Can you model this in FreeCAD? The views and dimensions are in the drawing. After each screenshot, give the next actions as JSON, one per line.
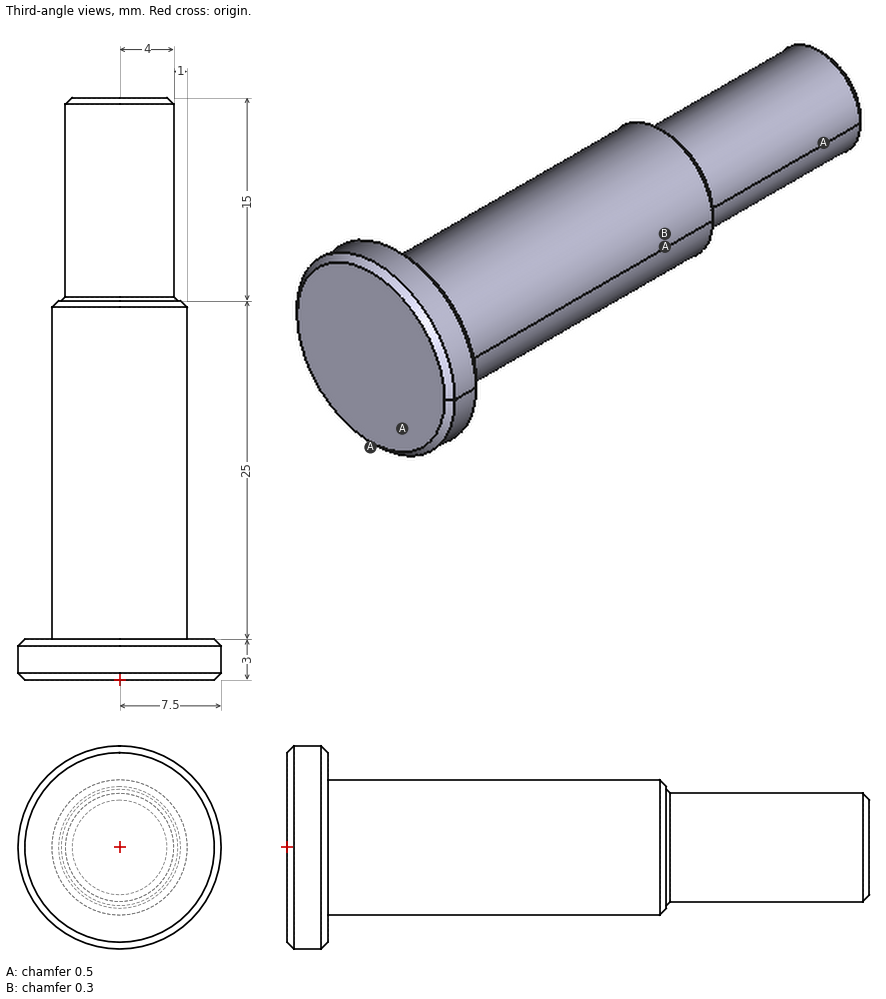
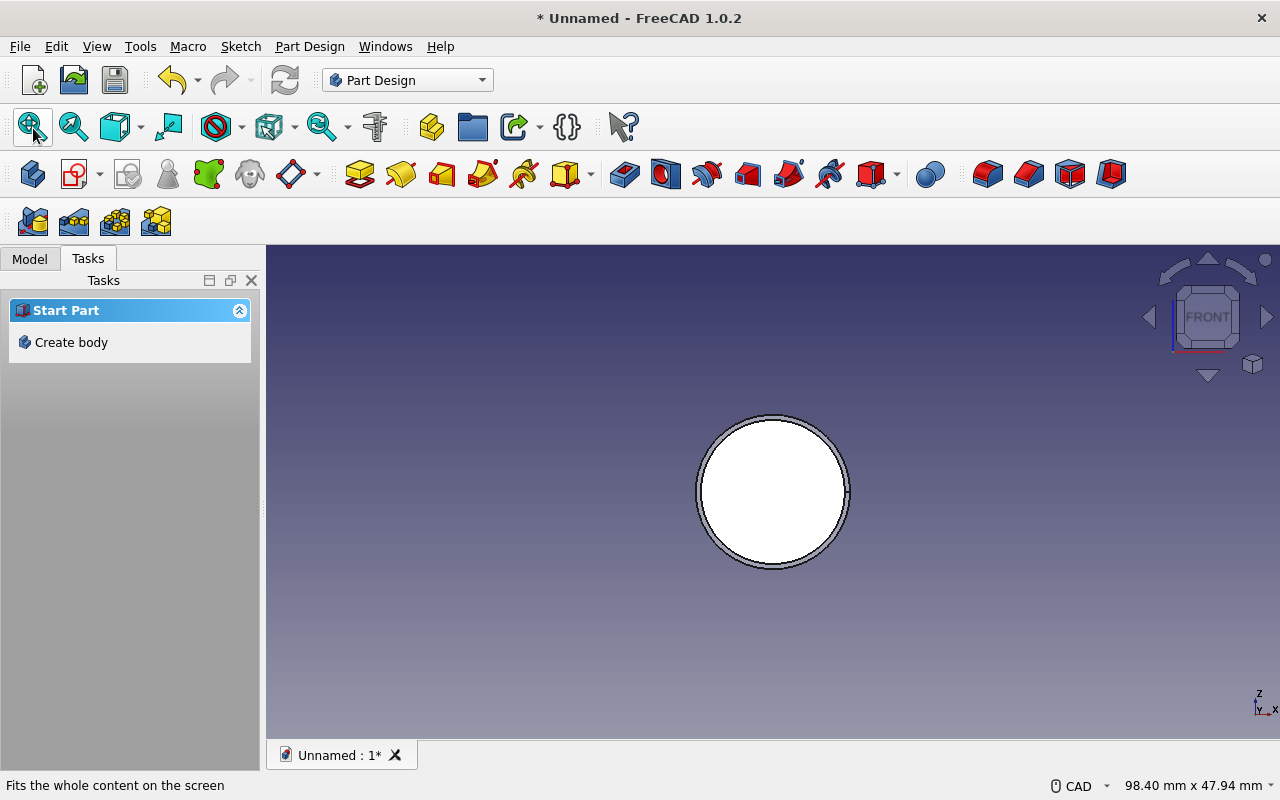
{"action": "key", "text": "3"}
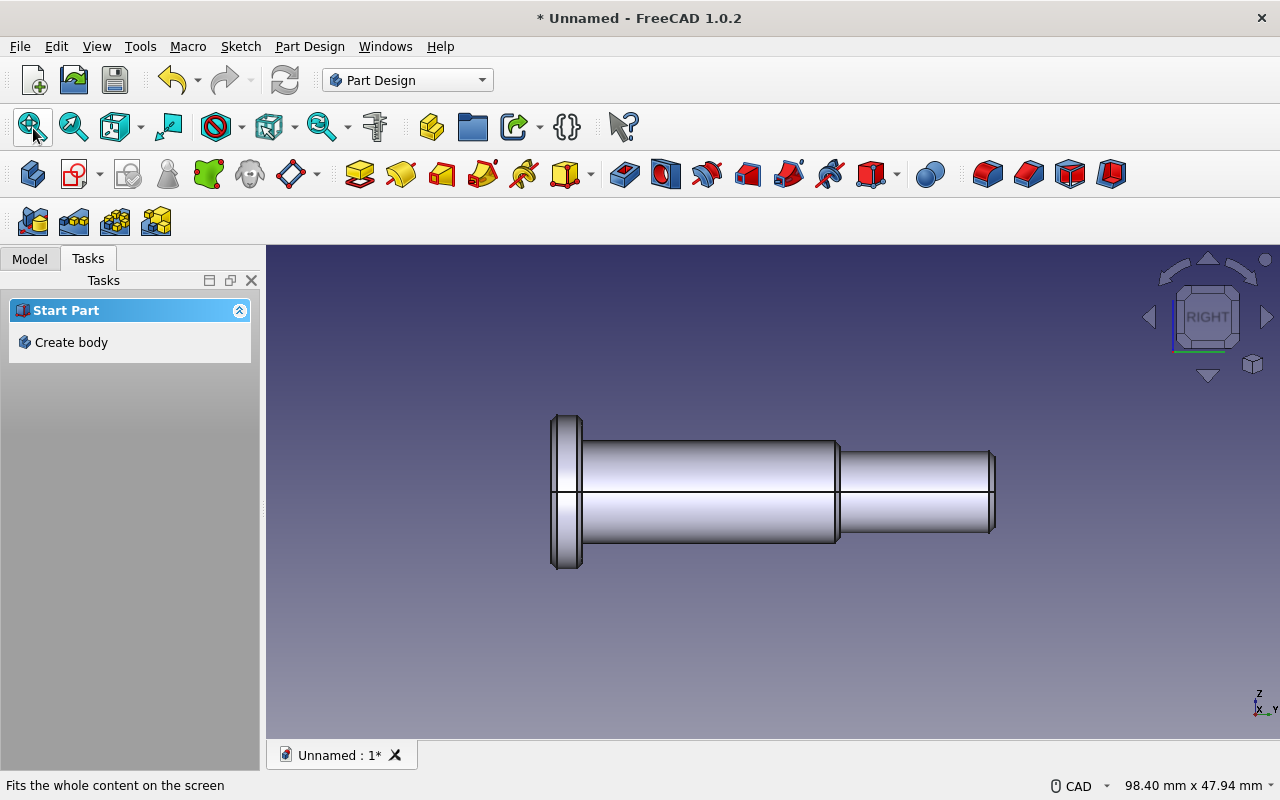
{"action": "left_click", "coordinate": [33, 128]}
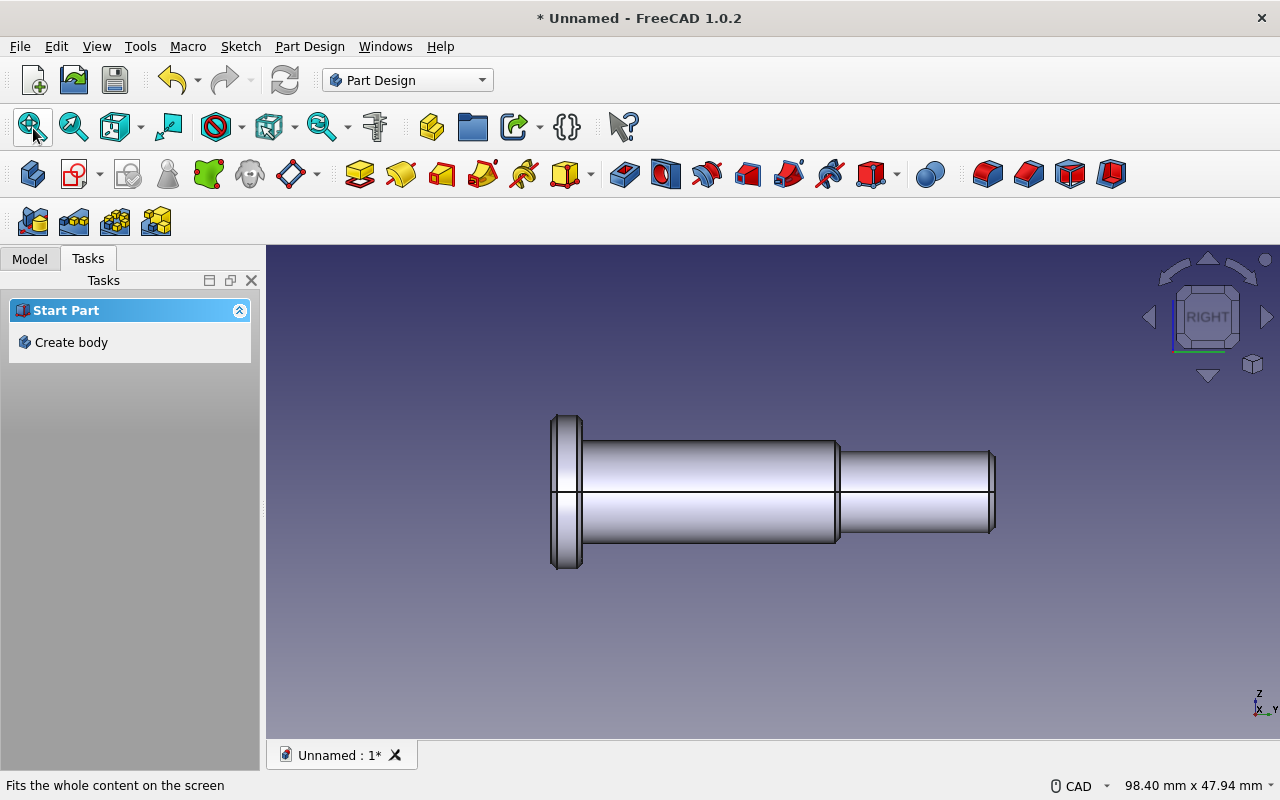
{"action": "key", "text": "5"}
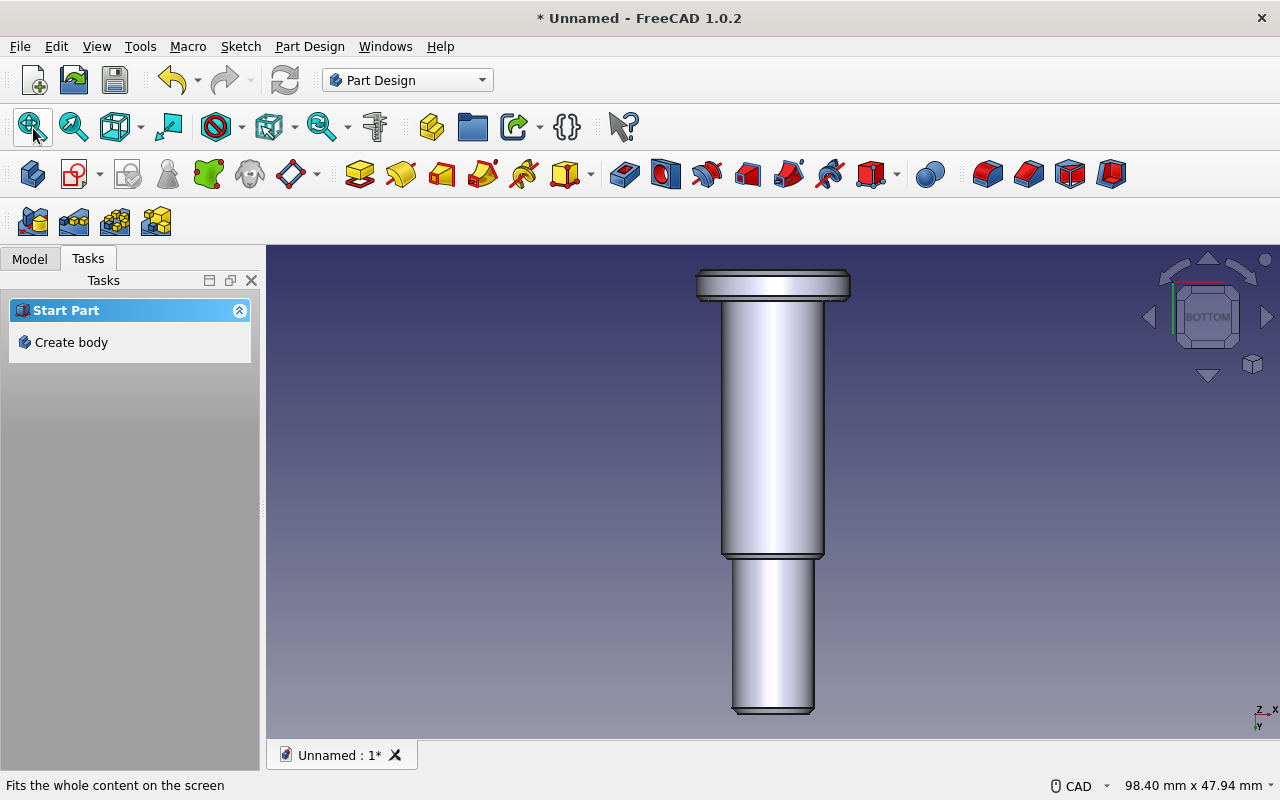
{"action": "key", "text": "4"}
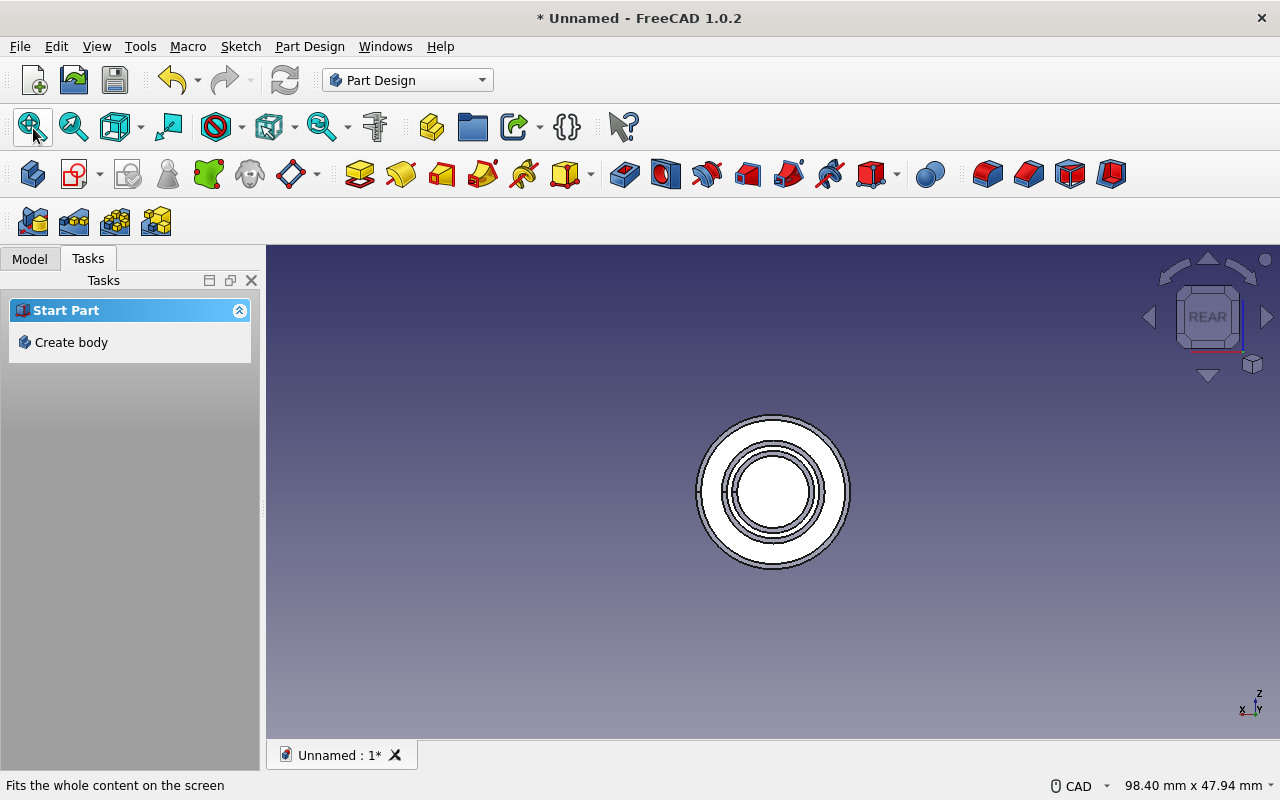
{"action": "left_click", "coordinate": [33, 128]}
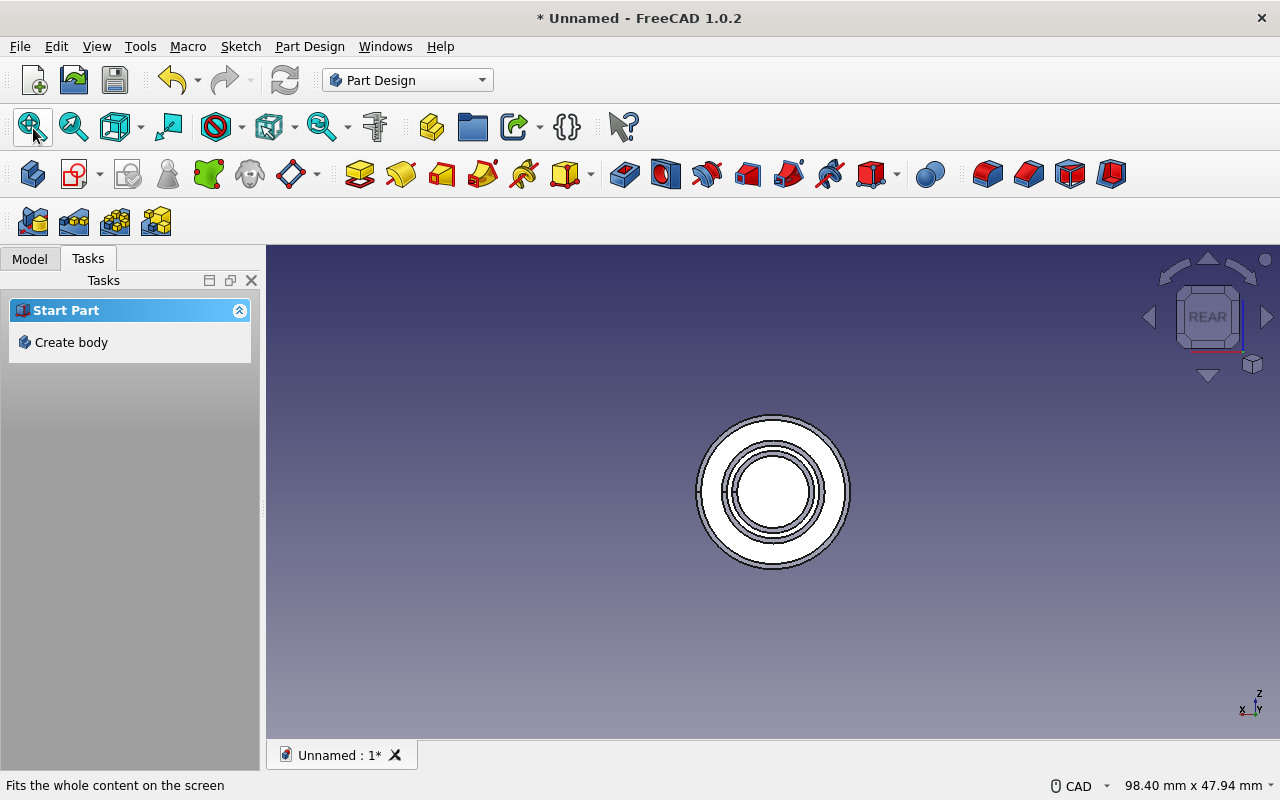
{"action": "key", "text": "6"}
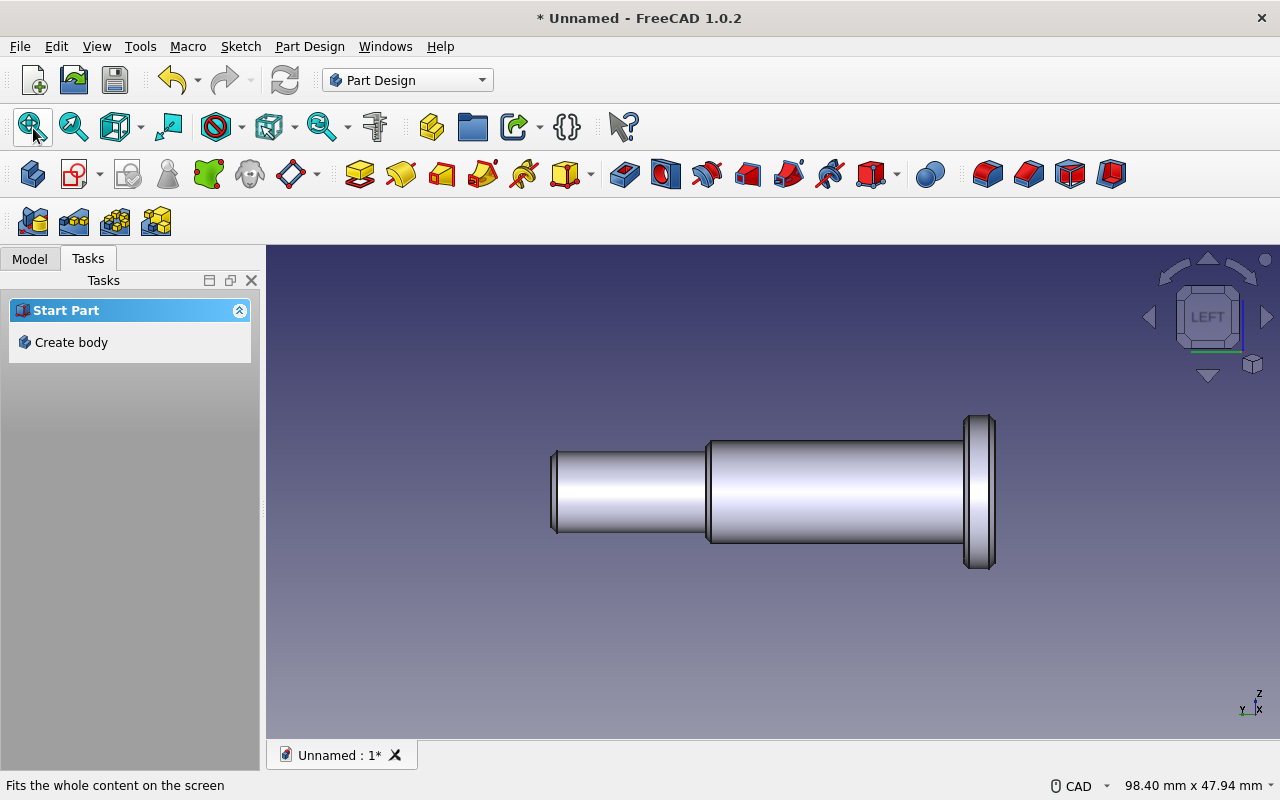
{"action": "left_click", "coordinate": [33, 128]}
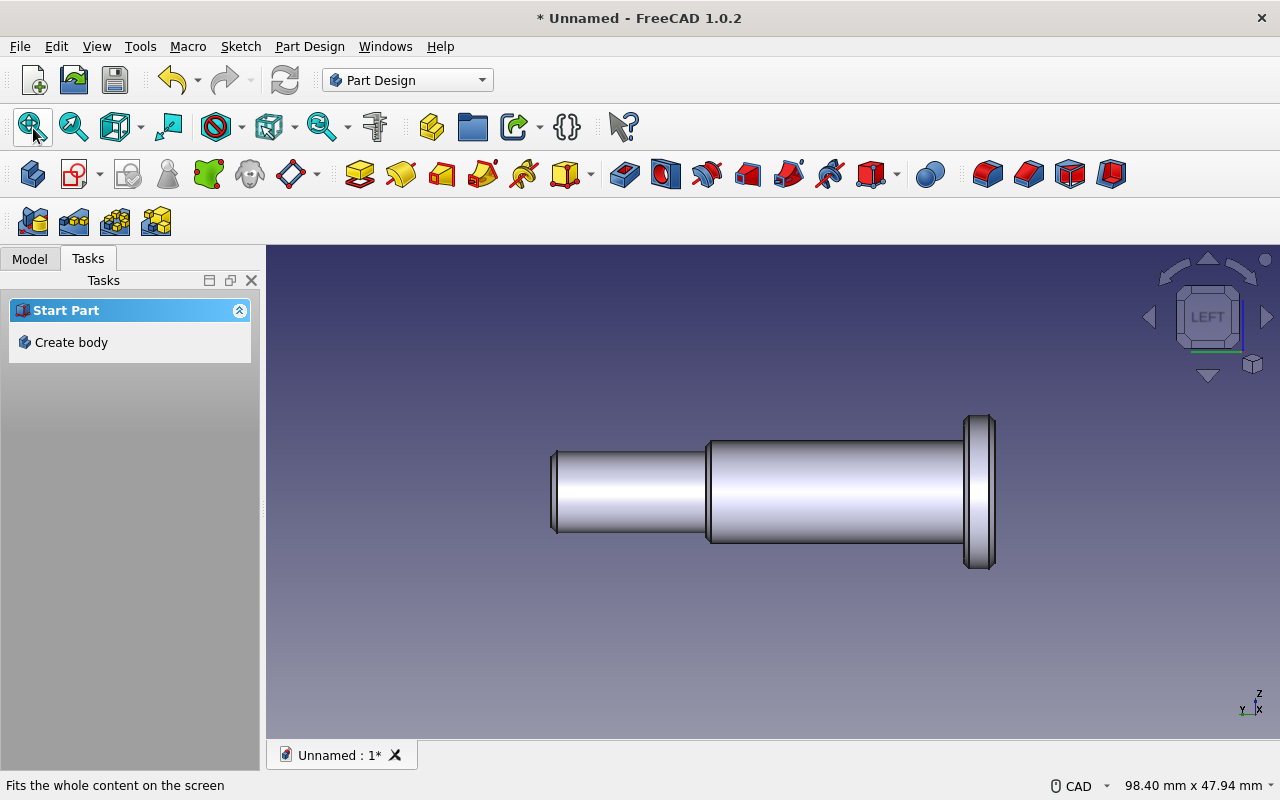
{"action": "key", "text": "v 3"}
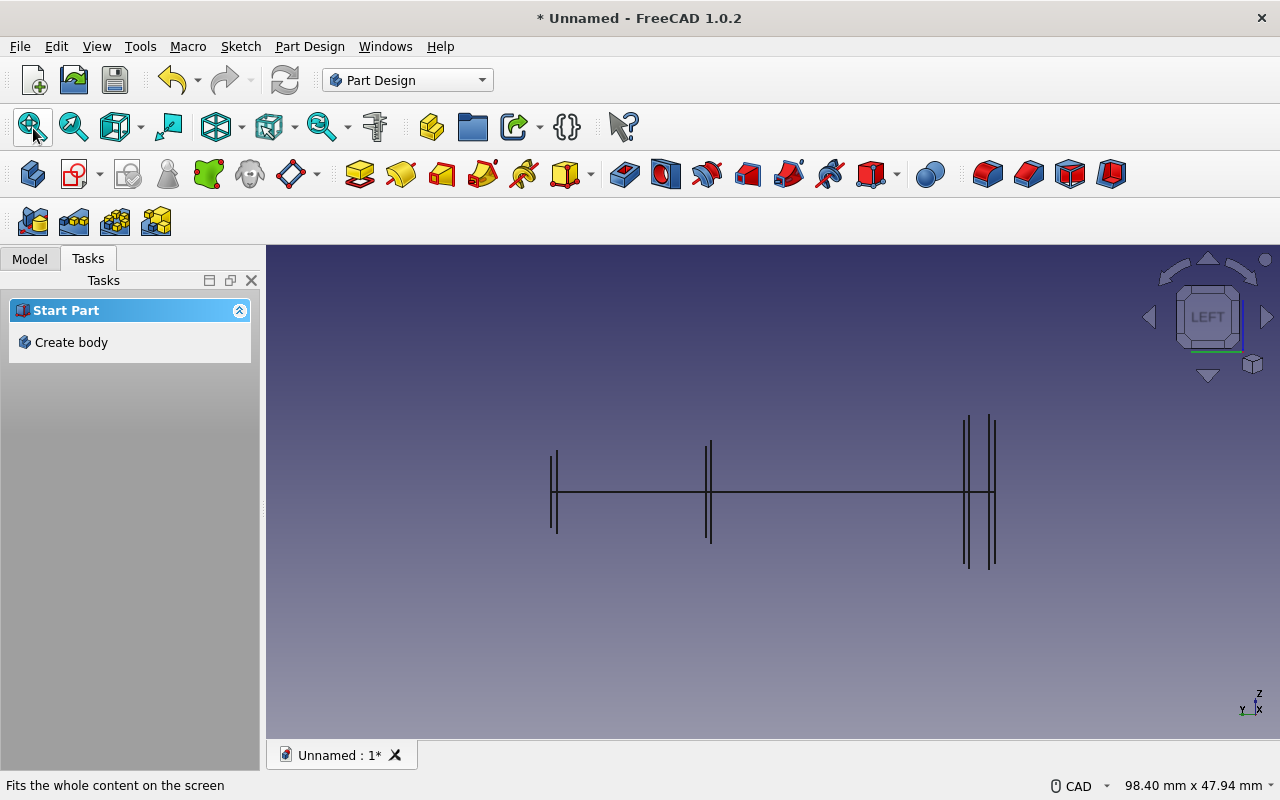
{"action": "key", "text": "0"}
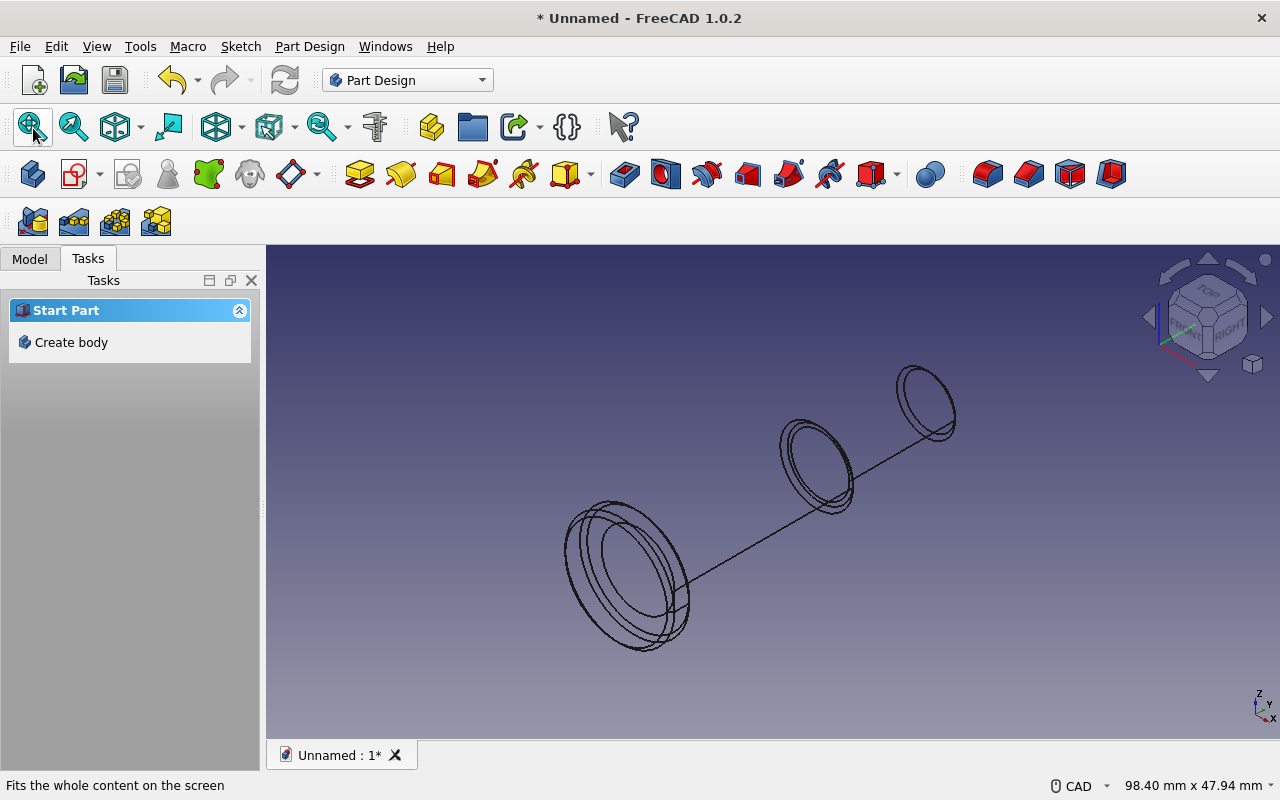
{"action": "left_click", "coordinate": [791, 447]}